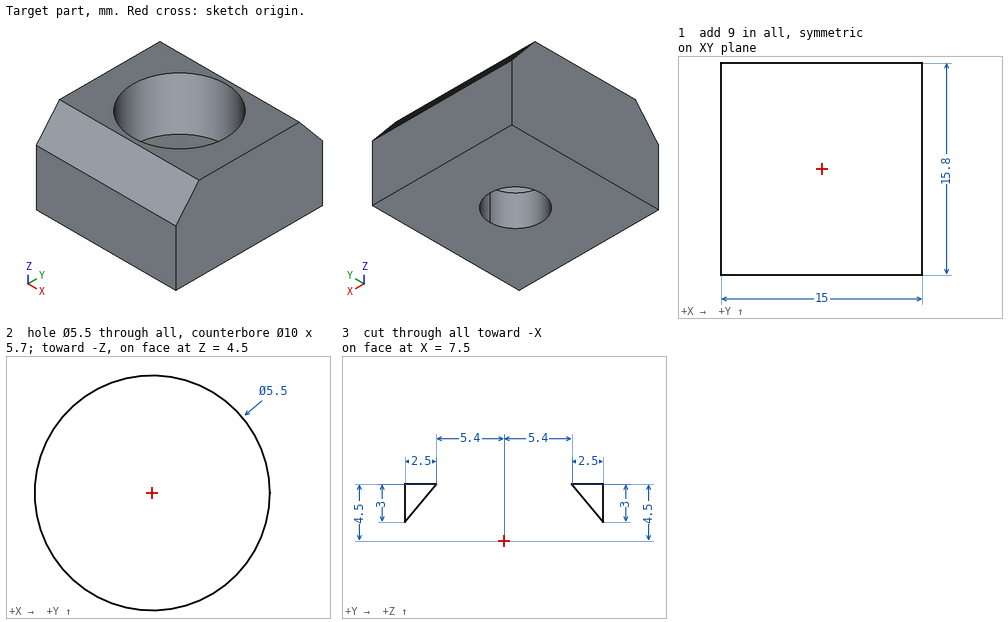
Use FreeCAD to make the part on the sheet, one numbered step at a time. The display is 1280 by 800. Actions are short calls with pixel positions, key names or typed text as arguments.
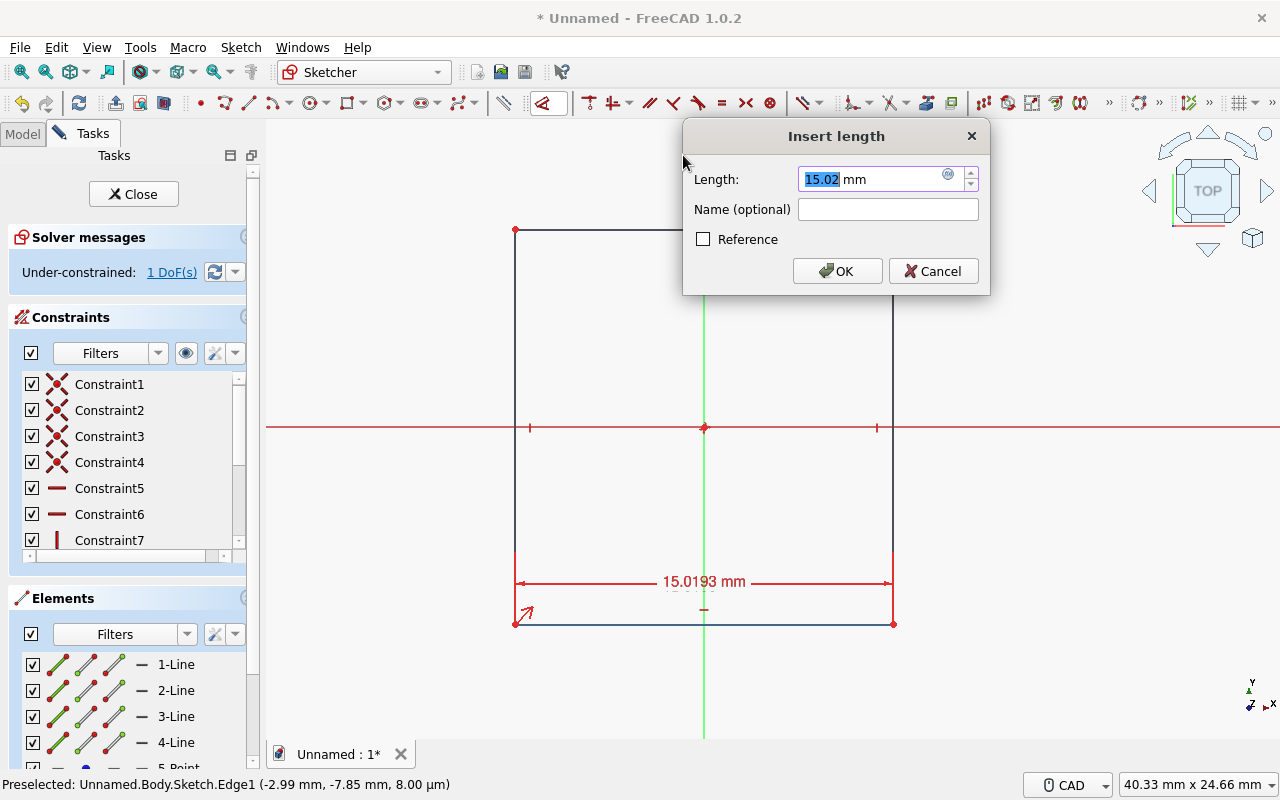
text(15)
key(Return)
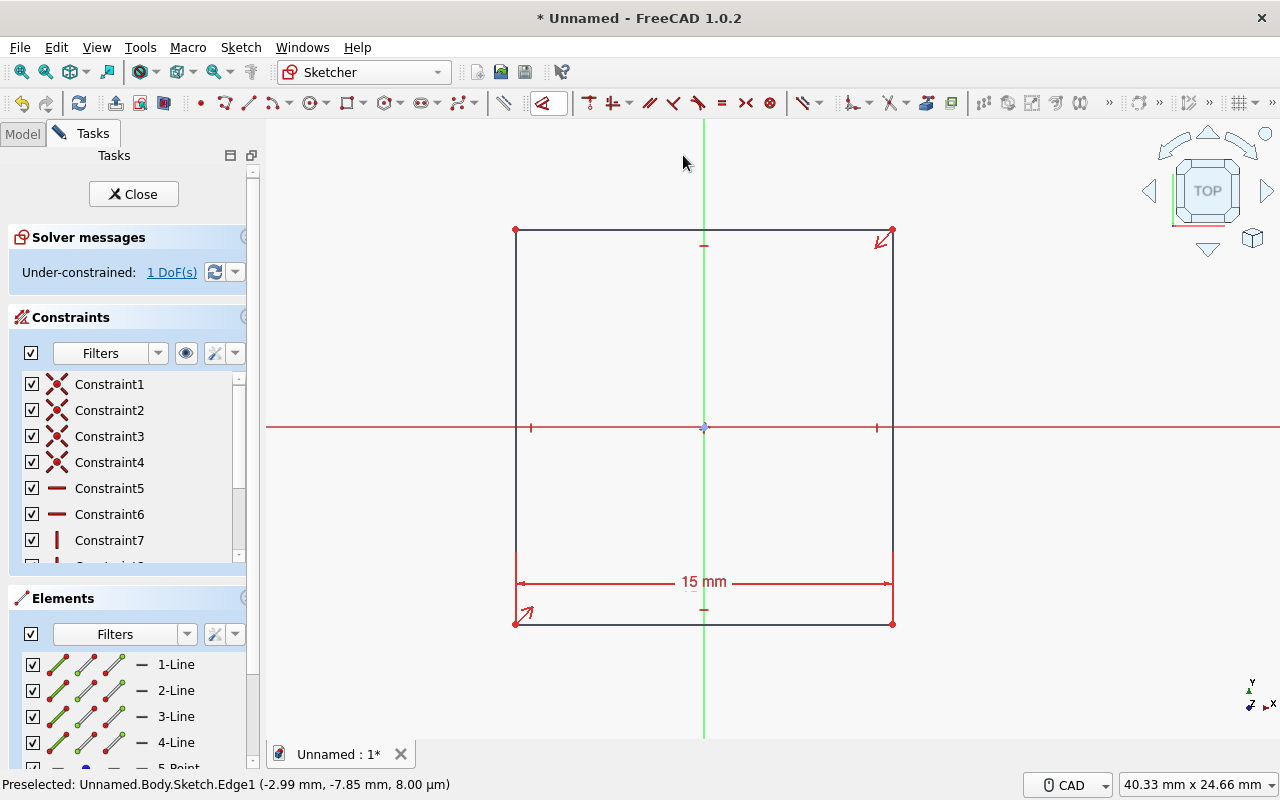
click(893, 506)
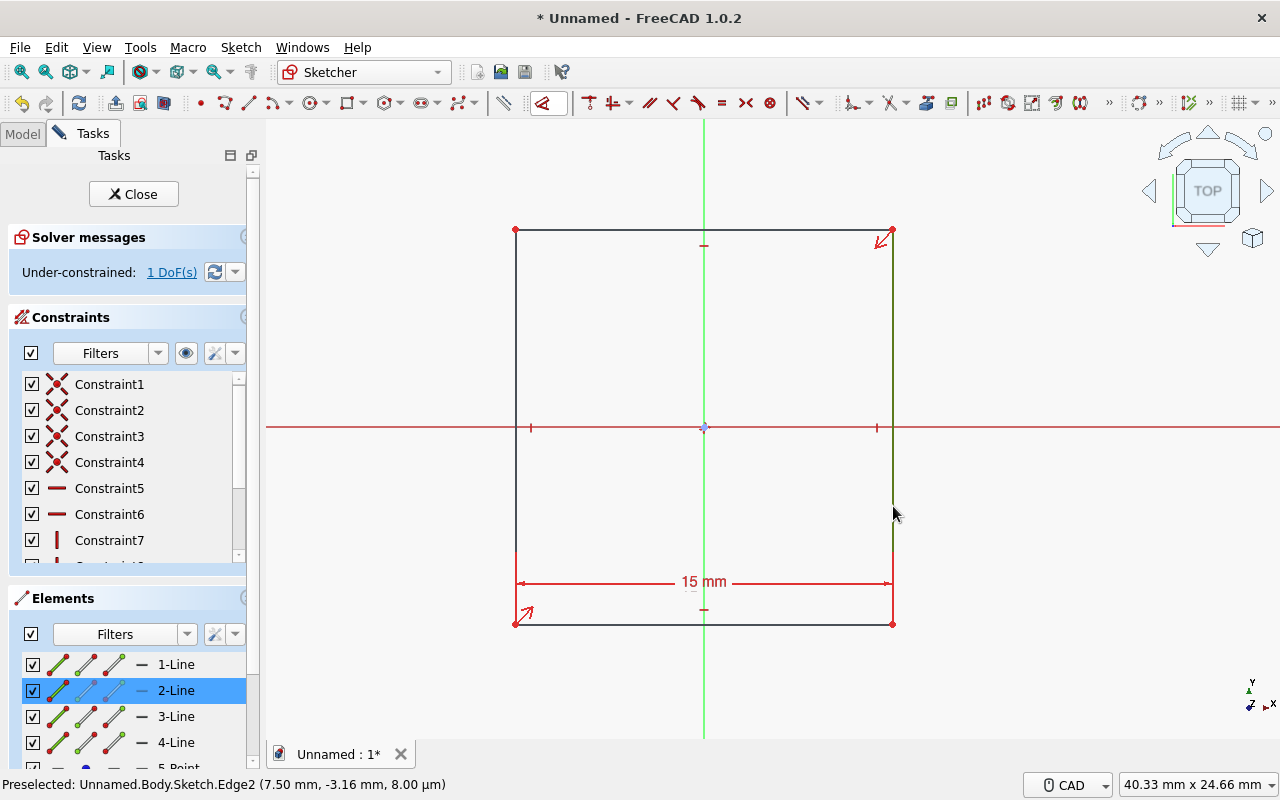
key(i)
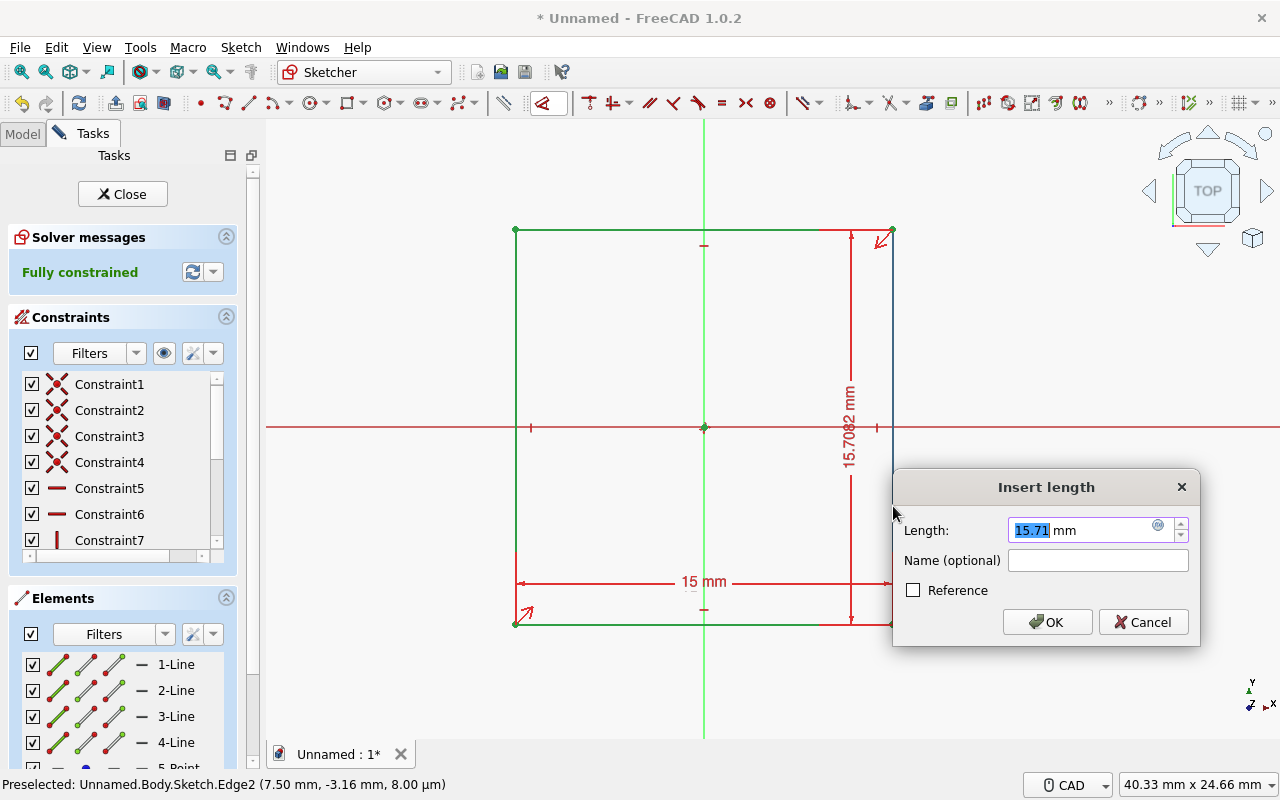
text(15.8)
key(Return)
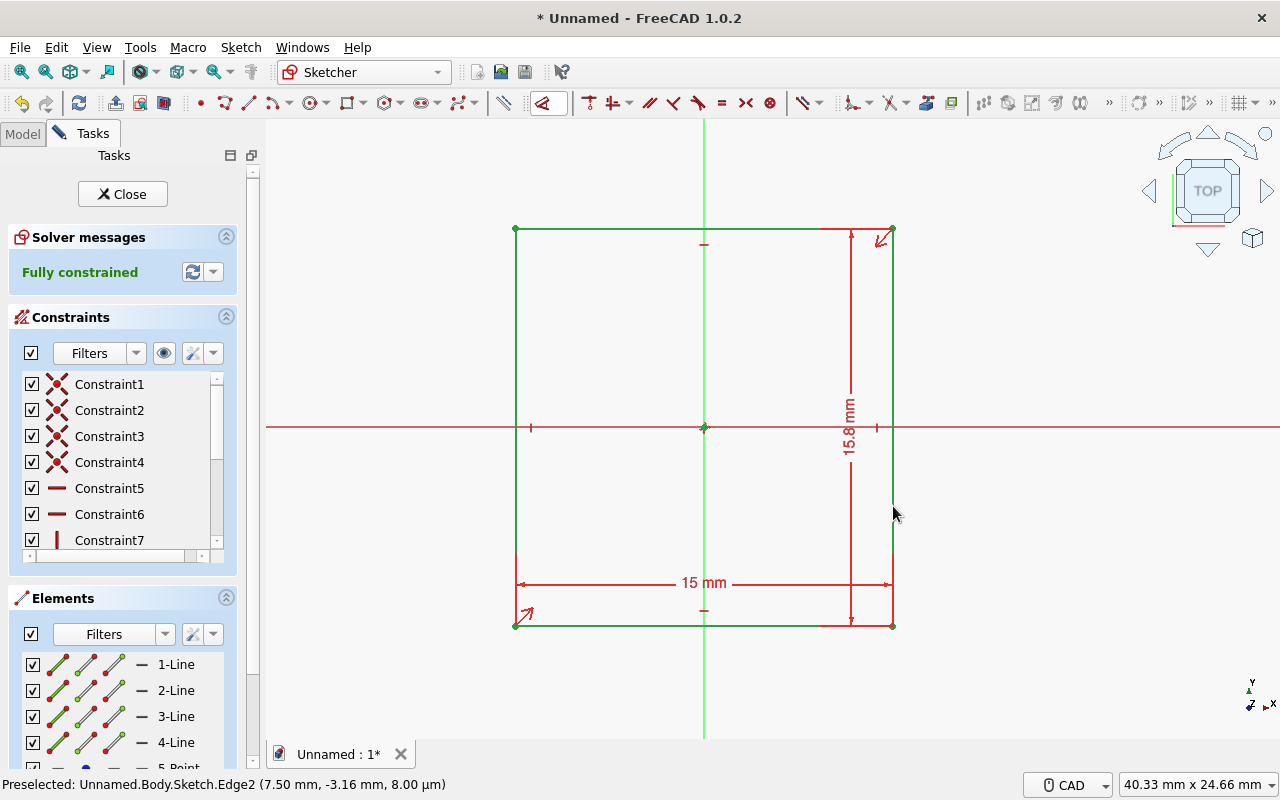
click(123, 194)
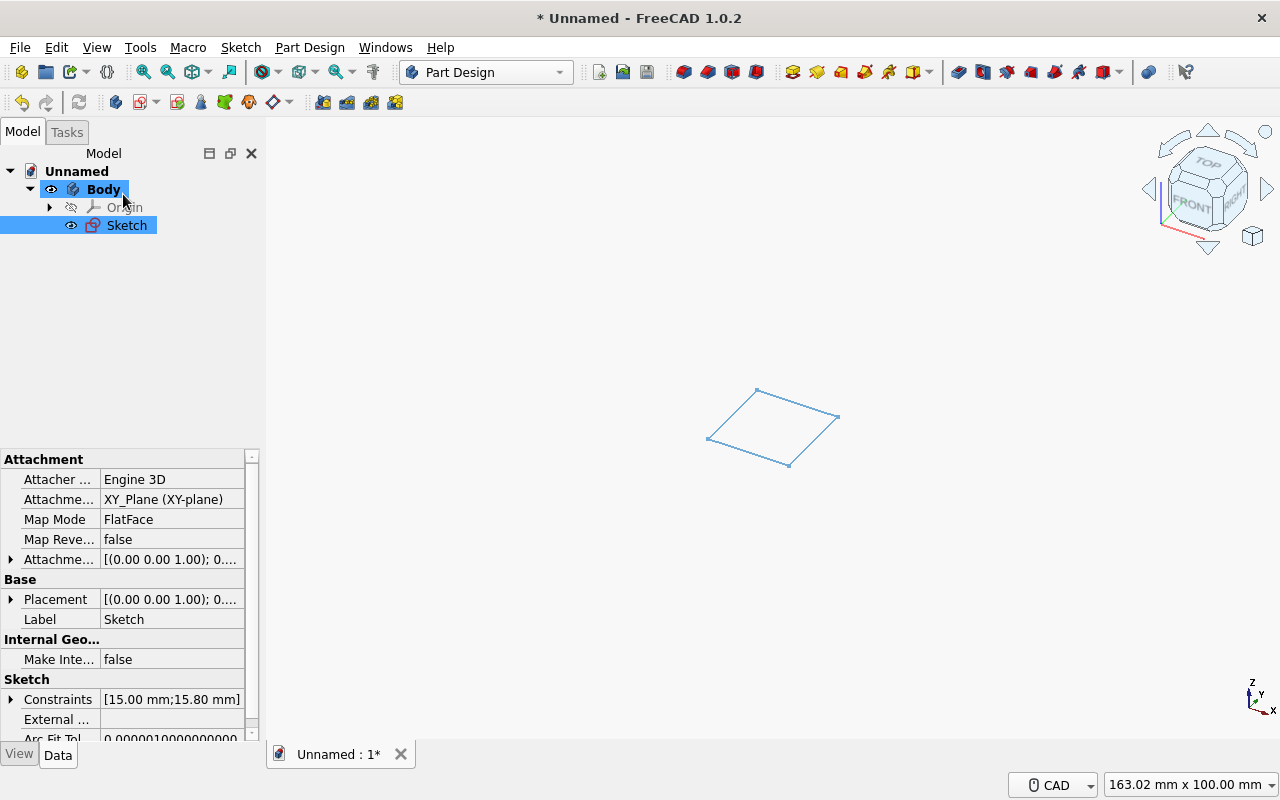
click(794, 72)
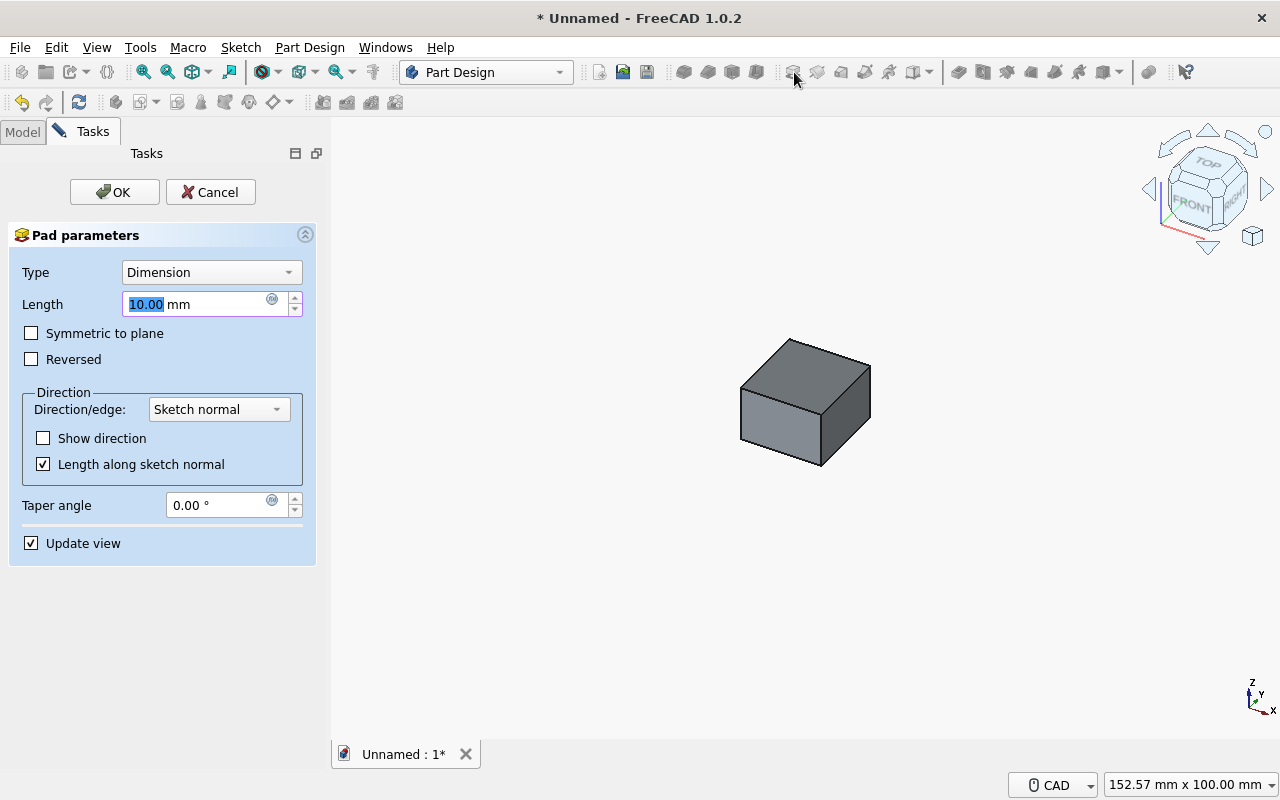
text(9)
key(Tab)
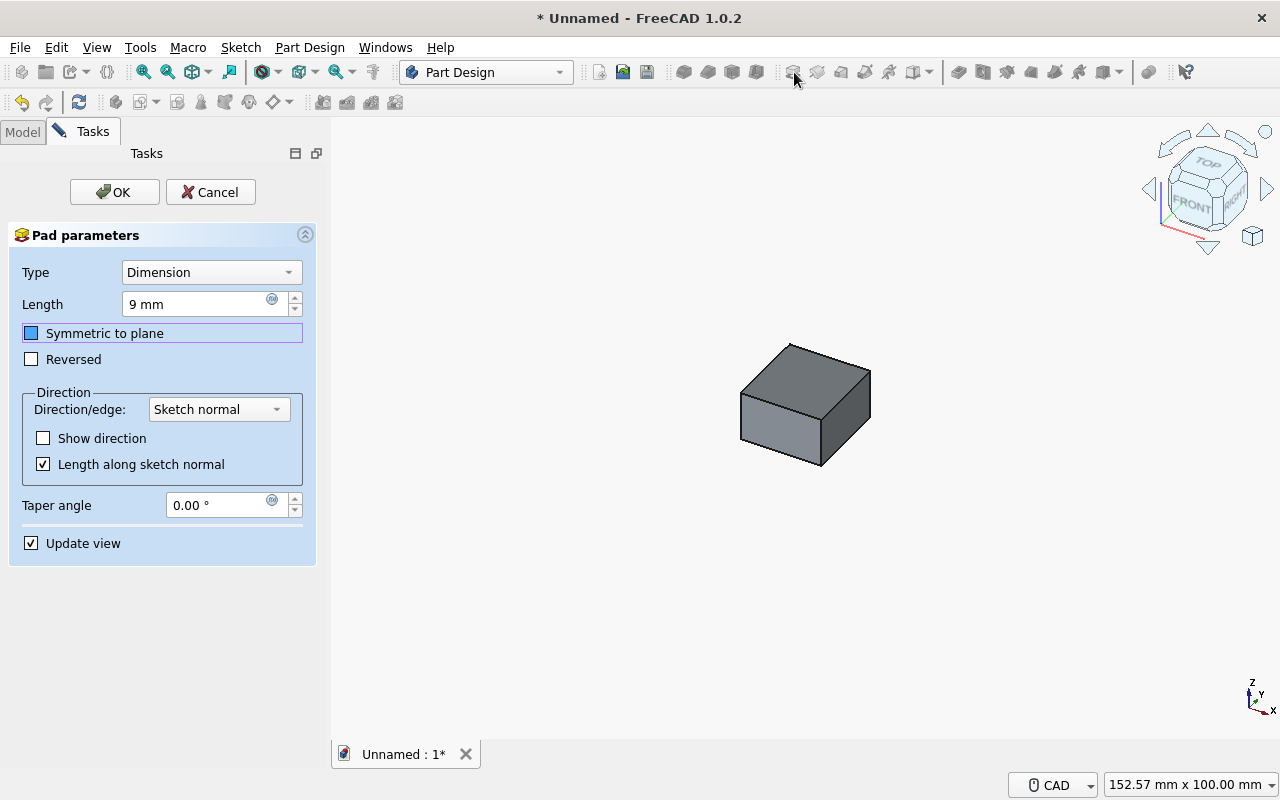
click(30, 333)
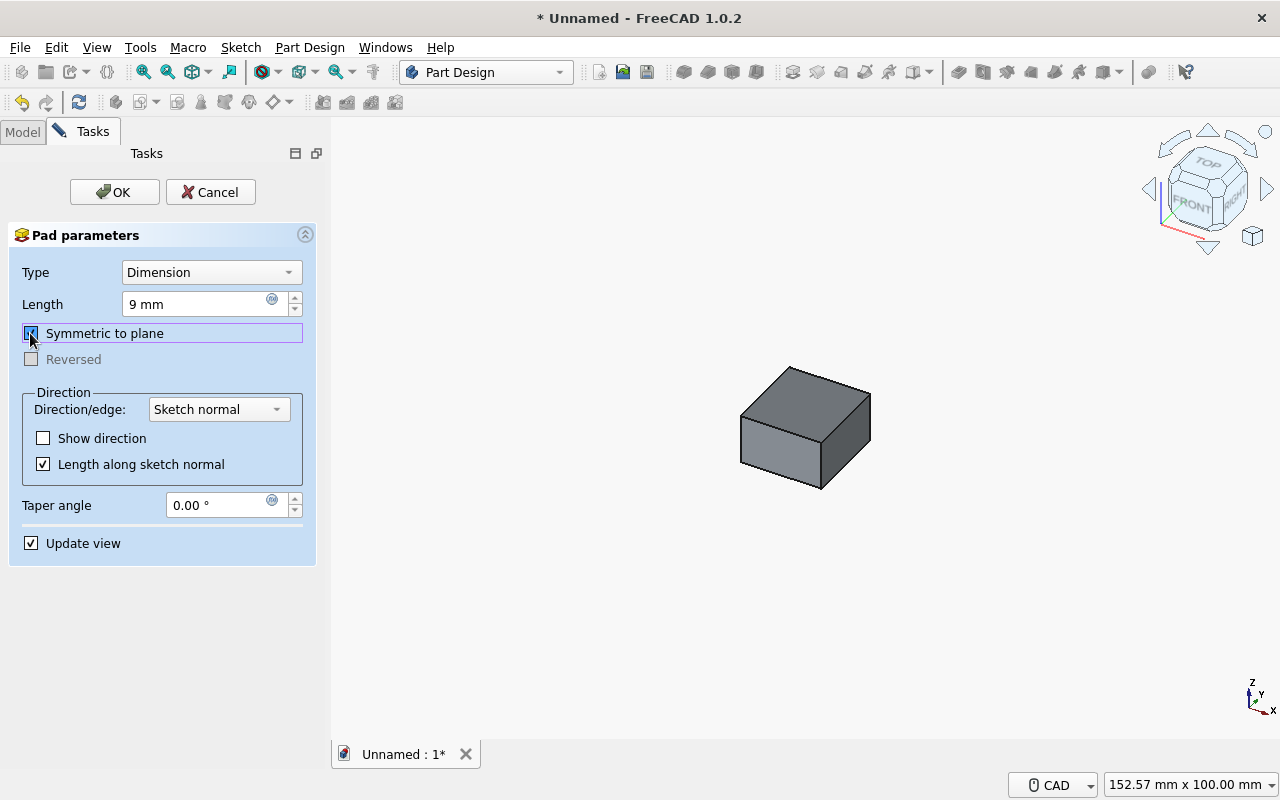
click(115, 192)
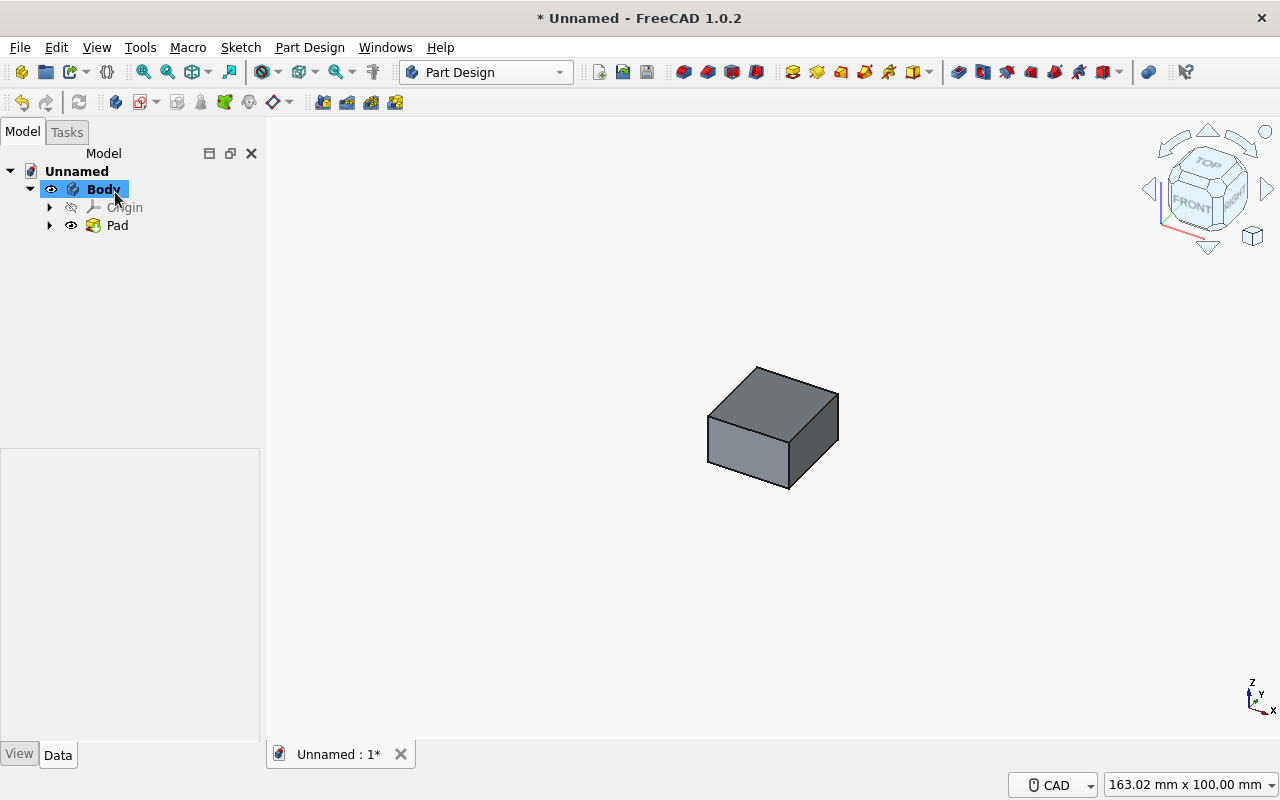
key(v)
key(f)